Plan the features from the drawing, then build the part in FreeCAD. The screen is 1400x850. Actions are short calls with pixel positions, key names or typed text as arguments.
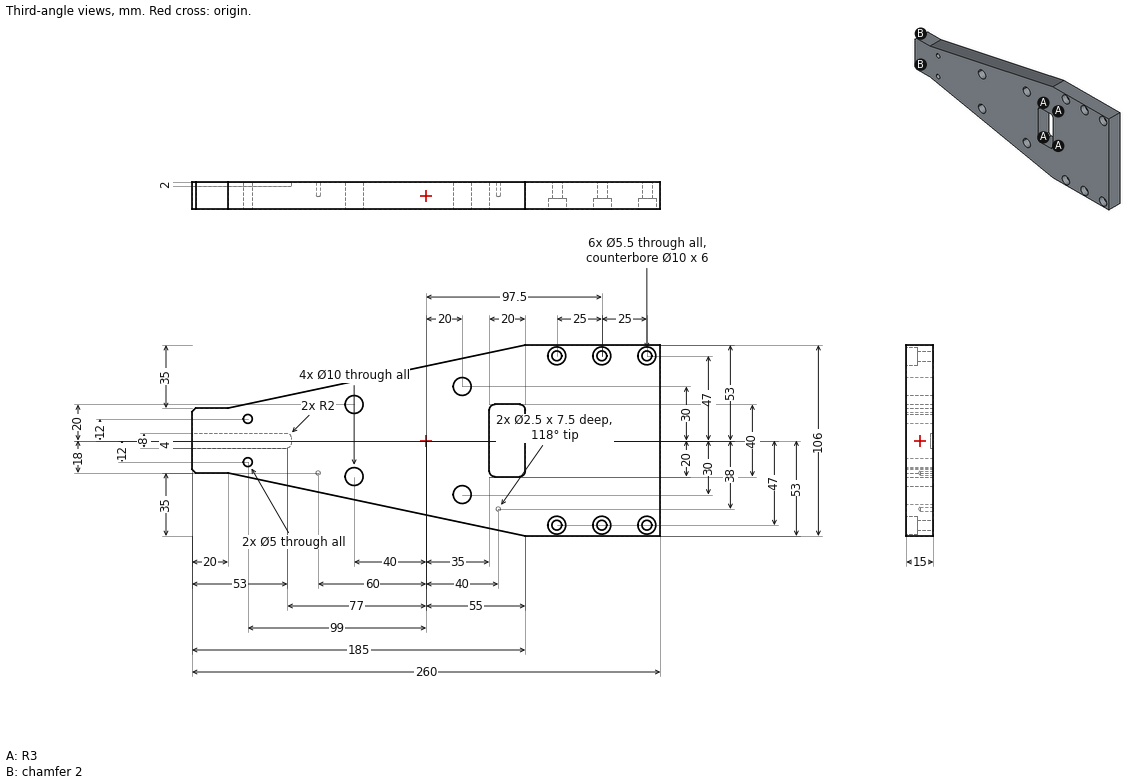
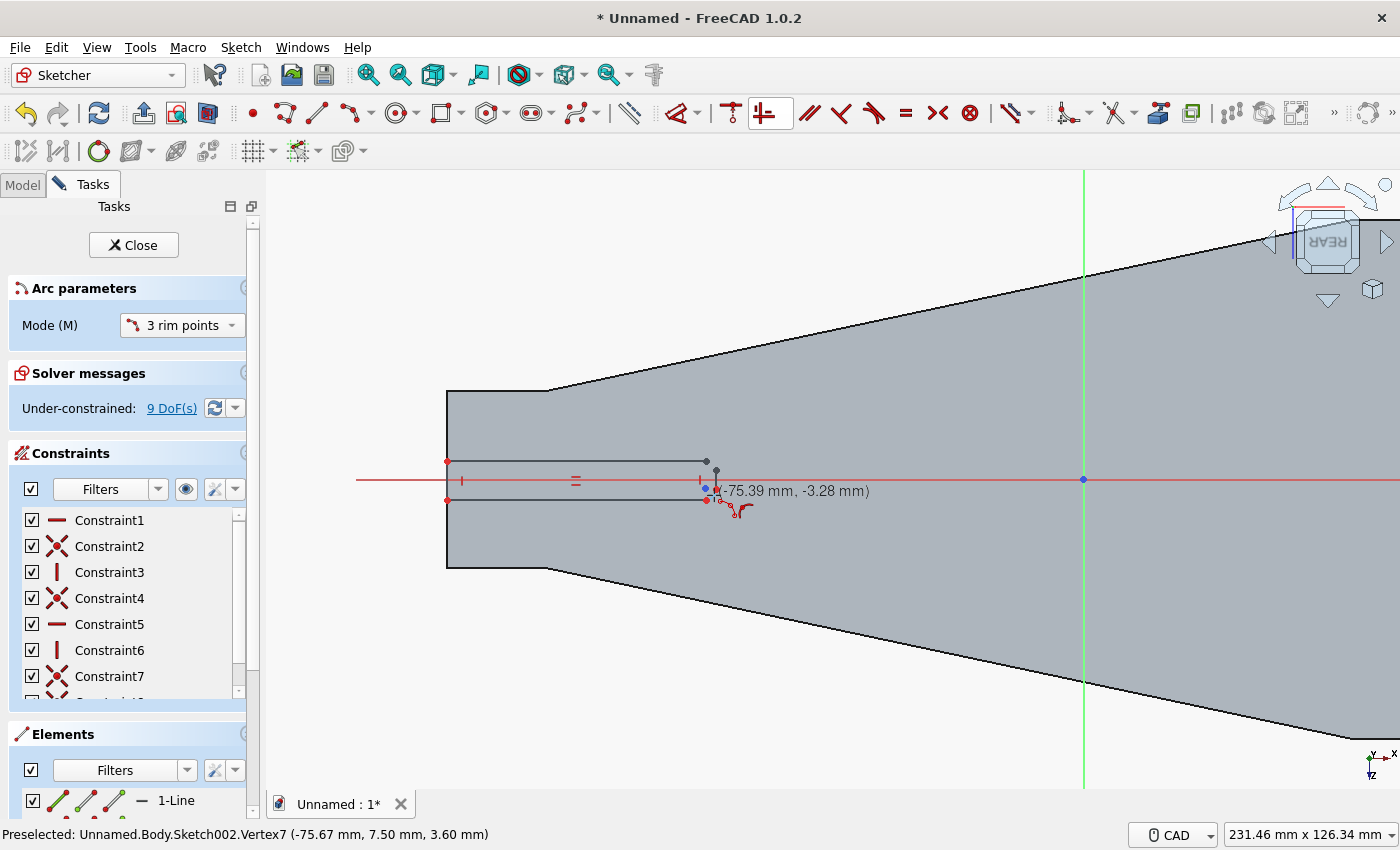
scroll(716, 470, up, 3)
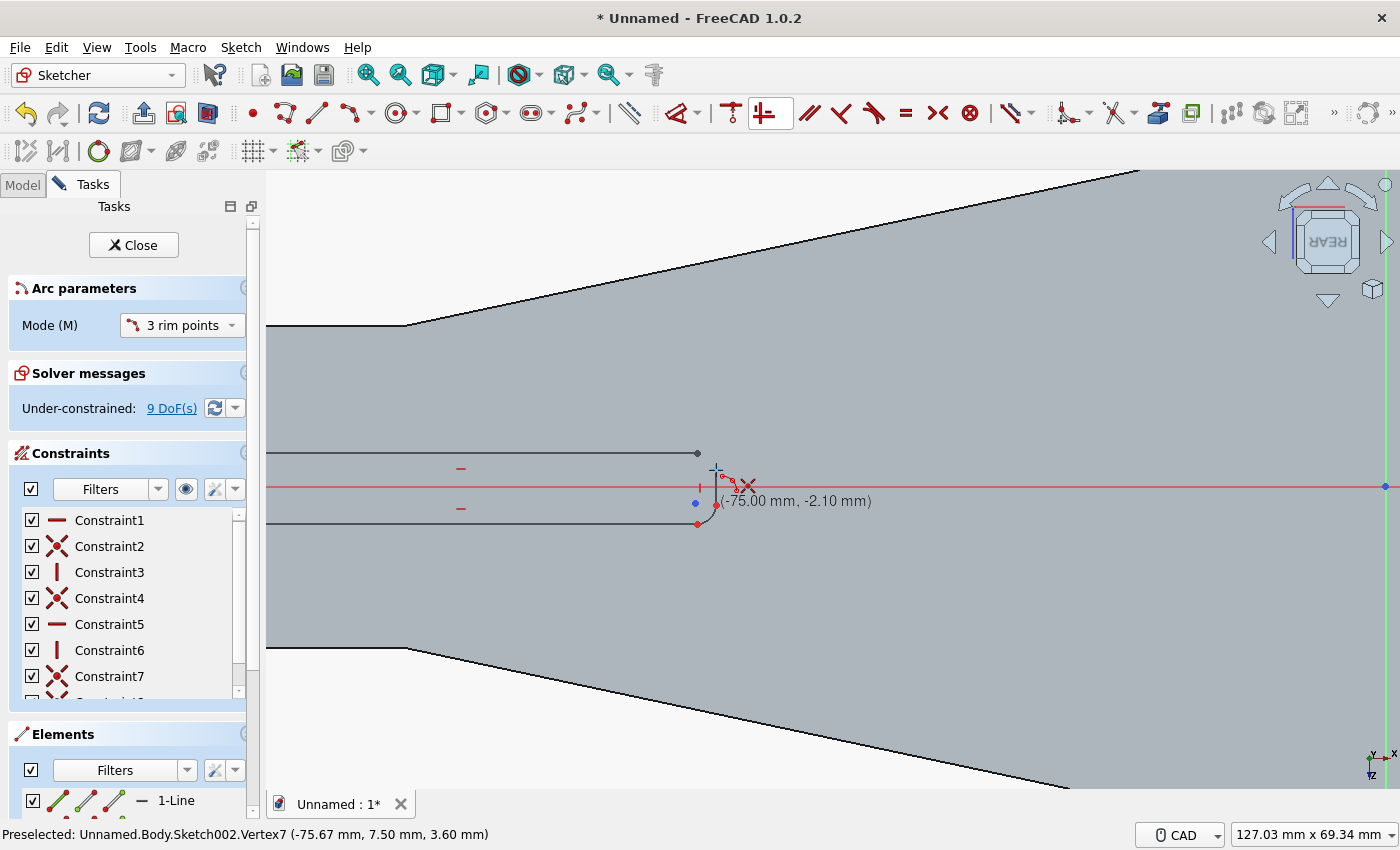
click(716, 470)
click(698, 453)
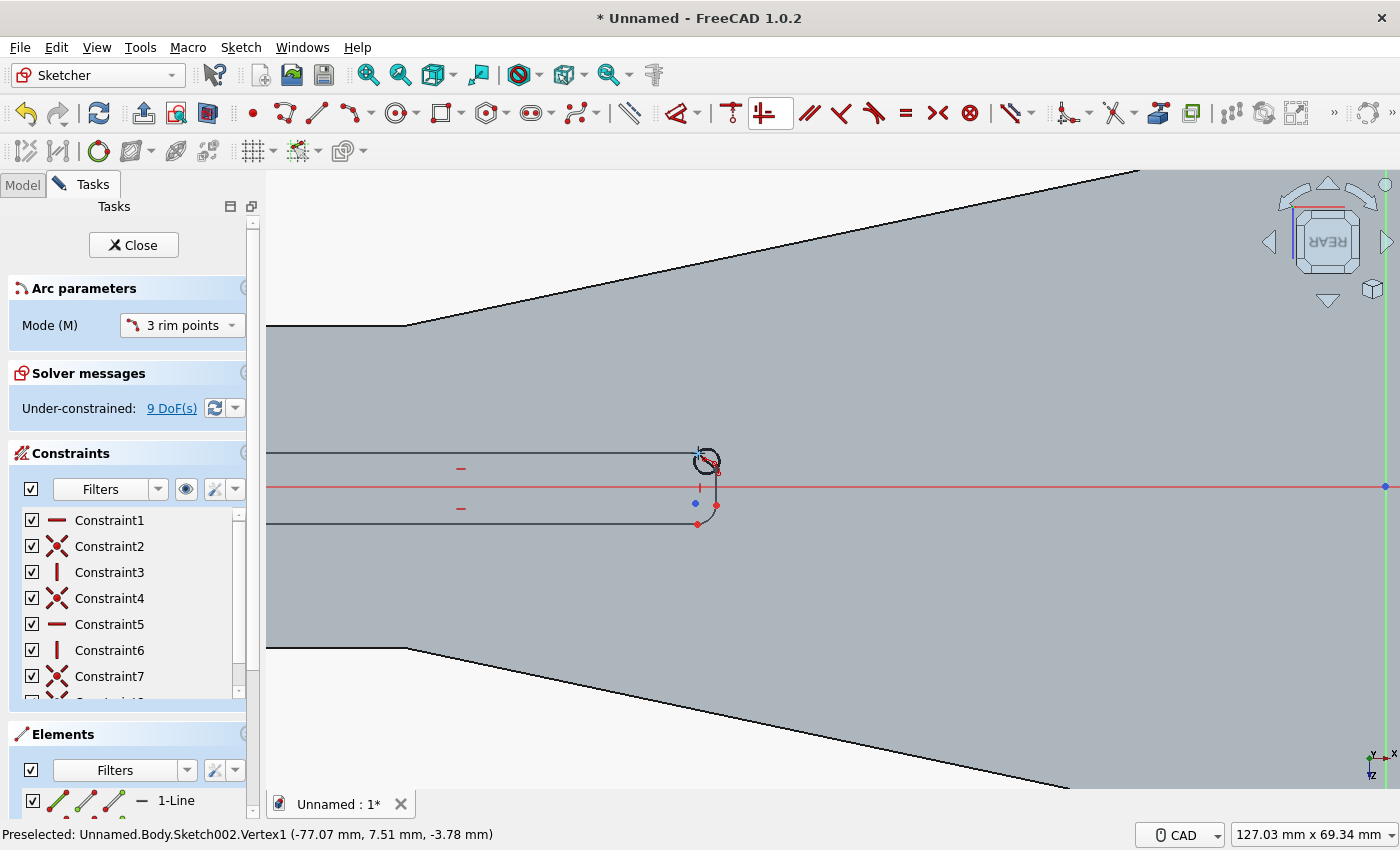
scroll(711, 456, up, 6)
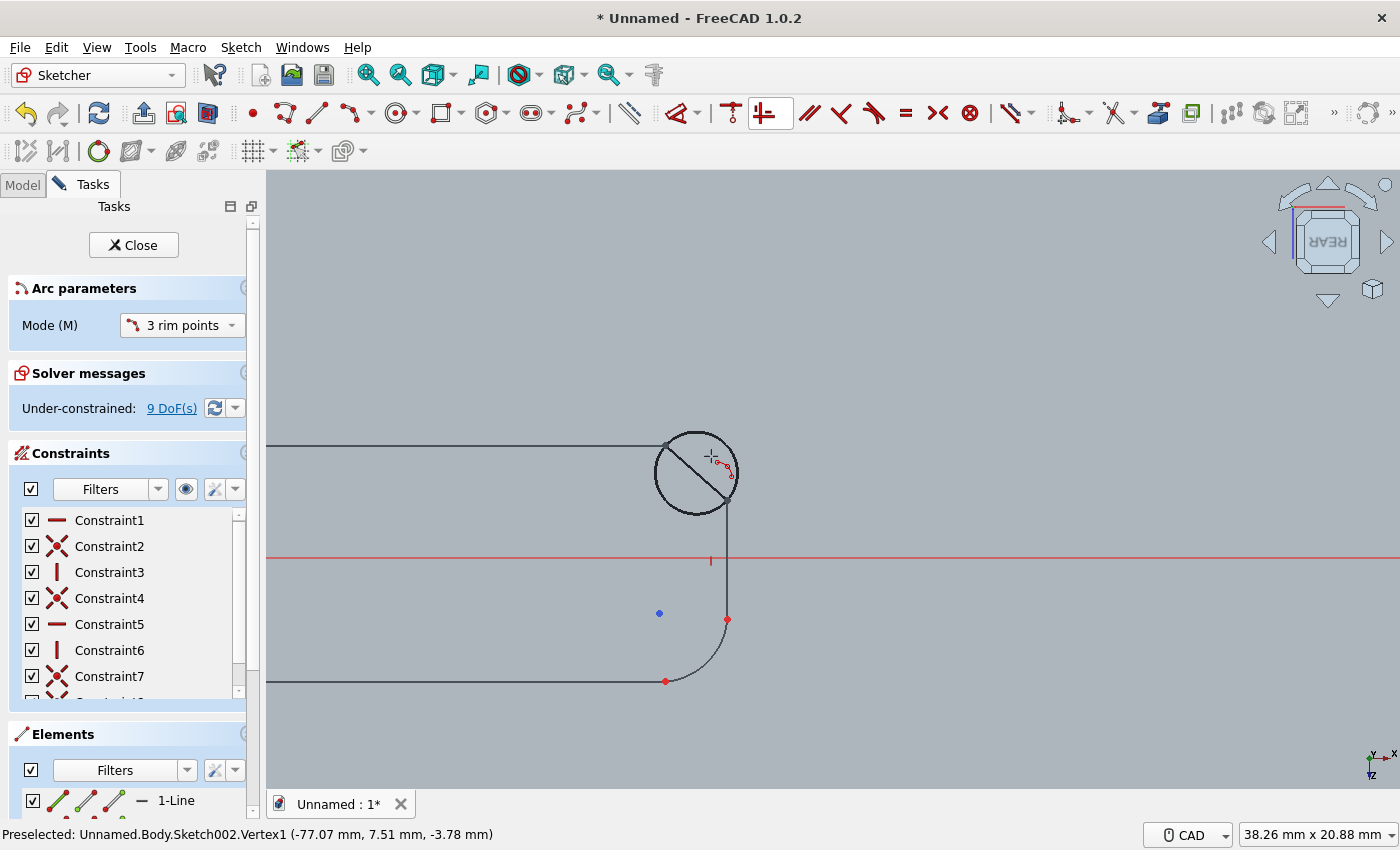
click(710, 456)
key(Escape)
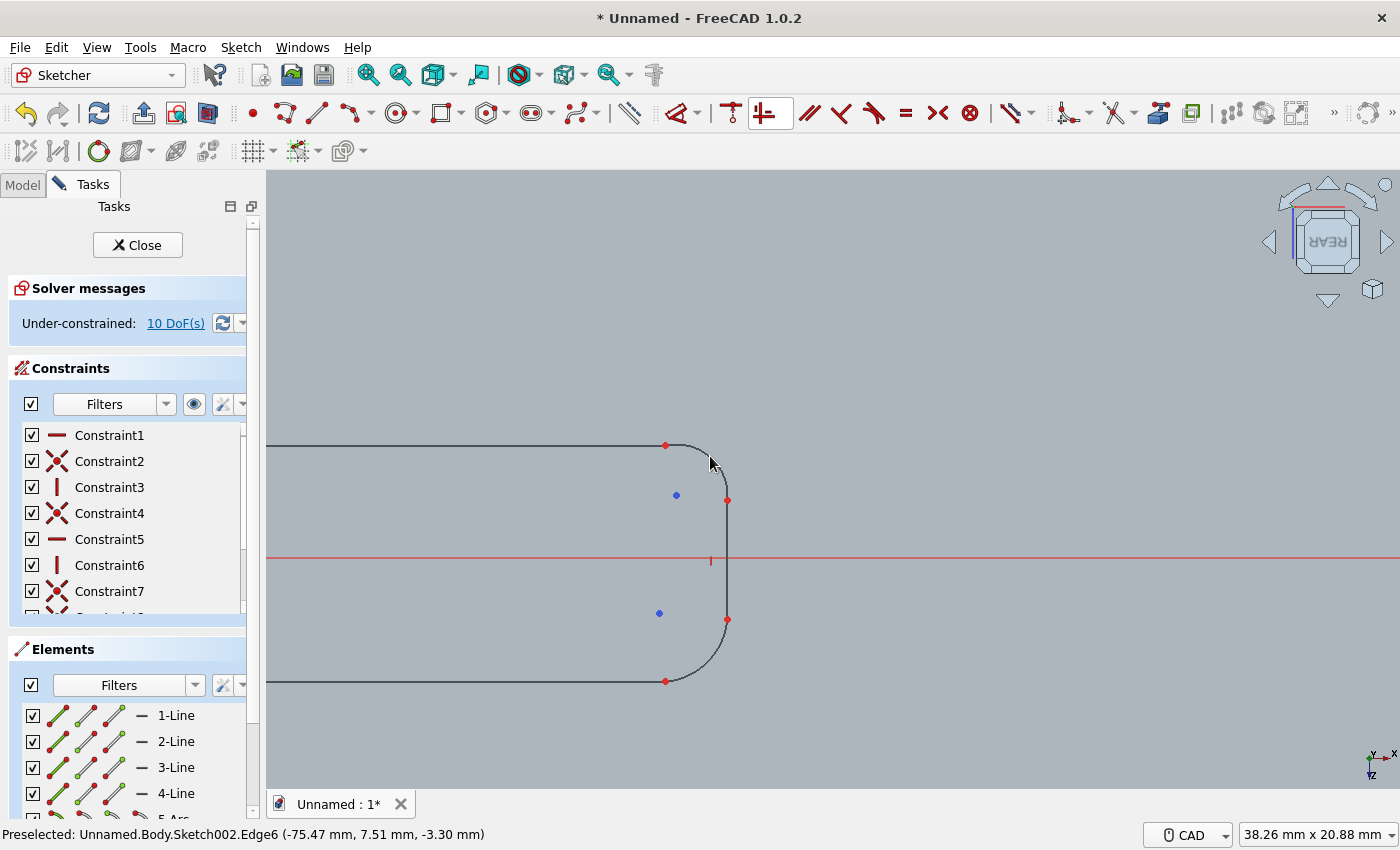
scroll(713, 464, down, 9)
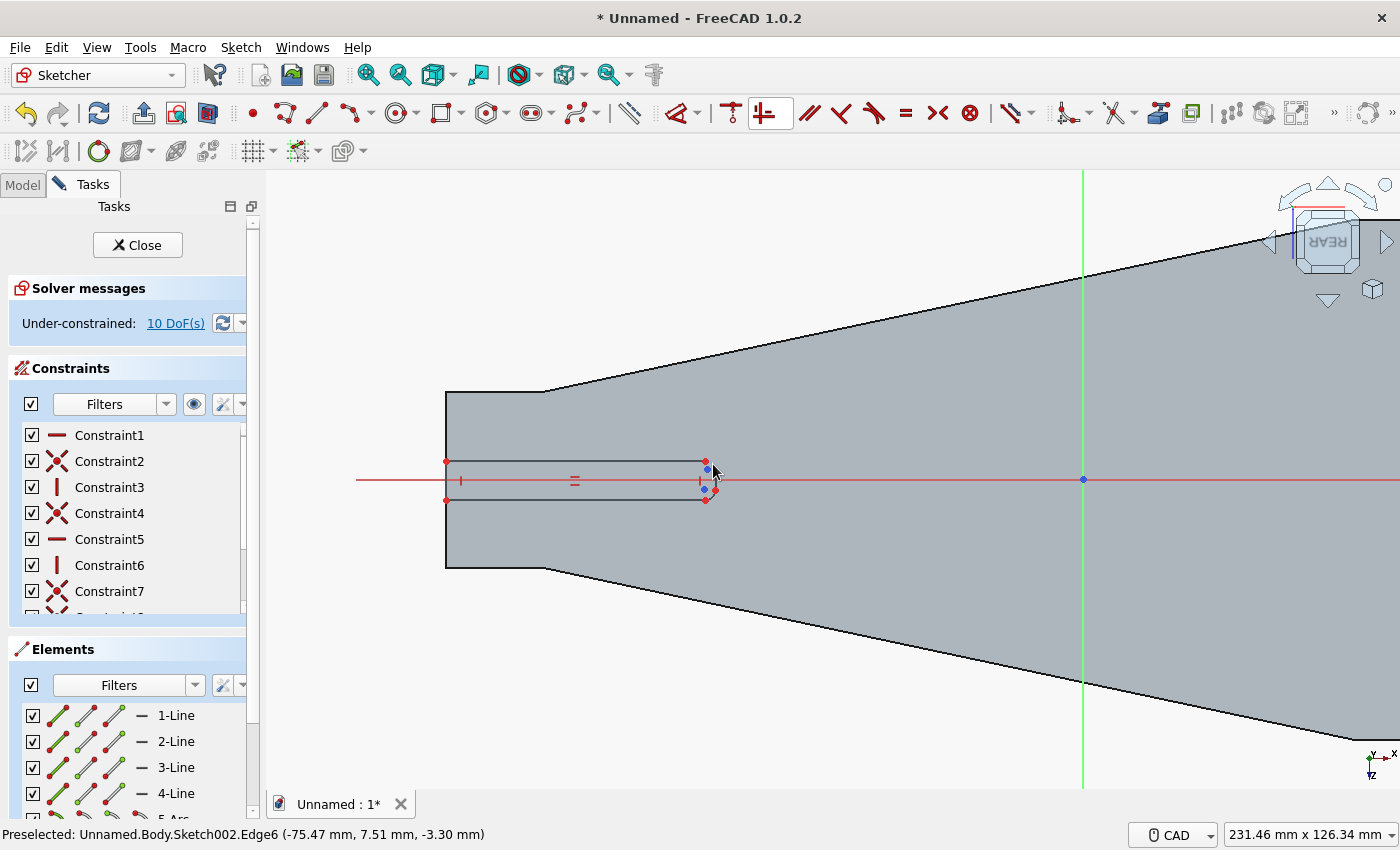
click(654, 461)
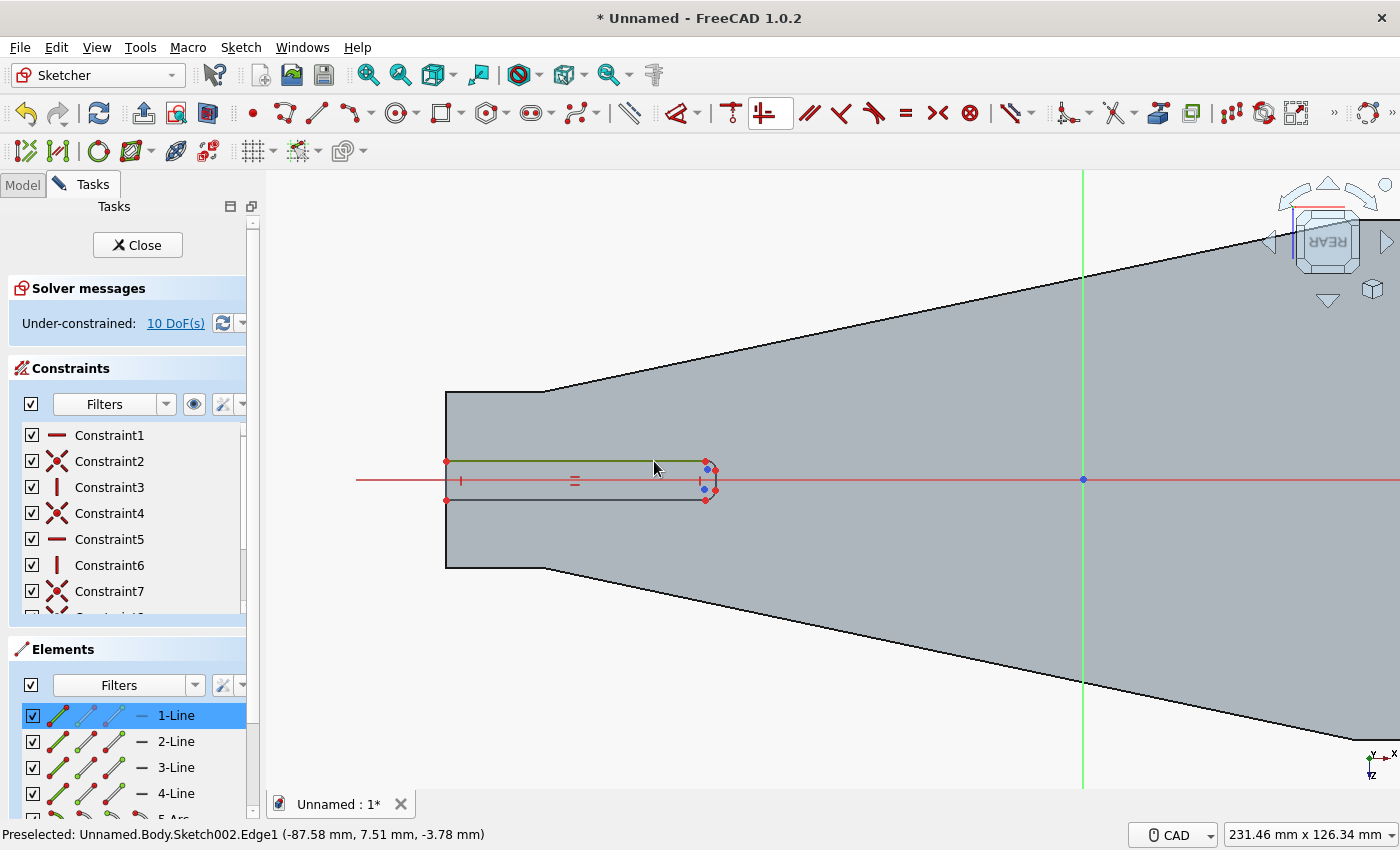
scroll(713, 463, up, 3)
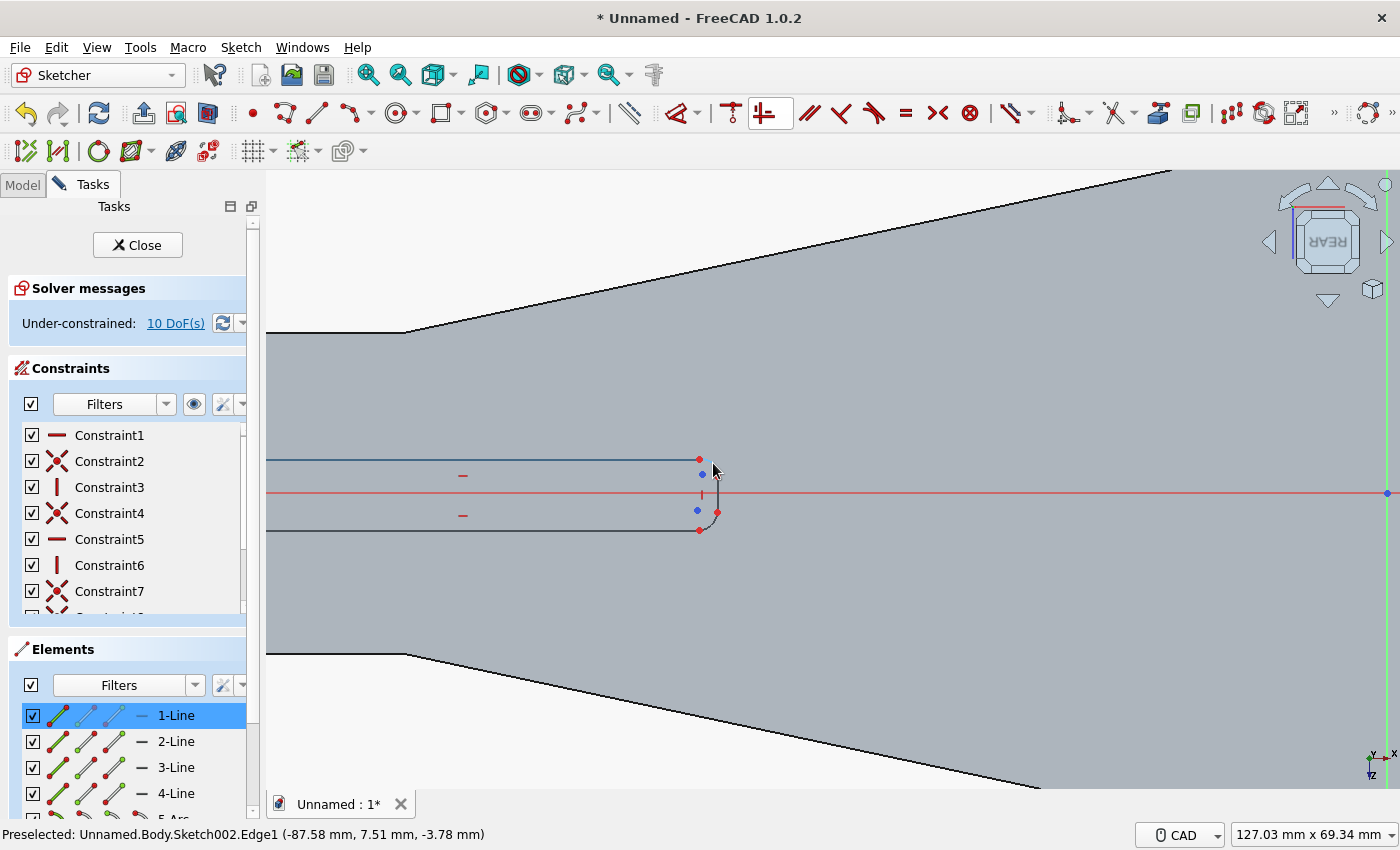
click(712, 463)